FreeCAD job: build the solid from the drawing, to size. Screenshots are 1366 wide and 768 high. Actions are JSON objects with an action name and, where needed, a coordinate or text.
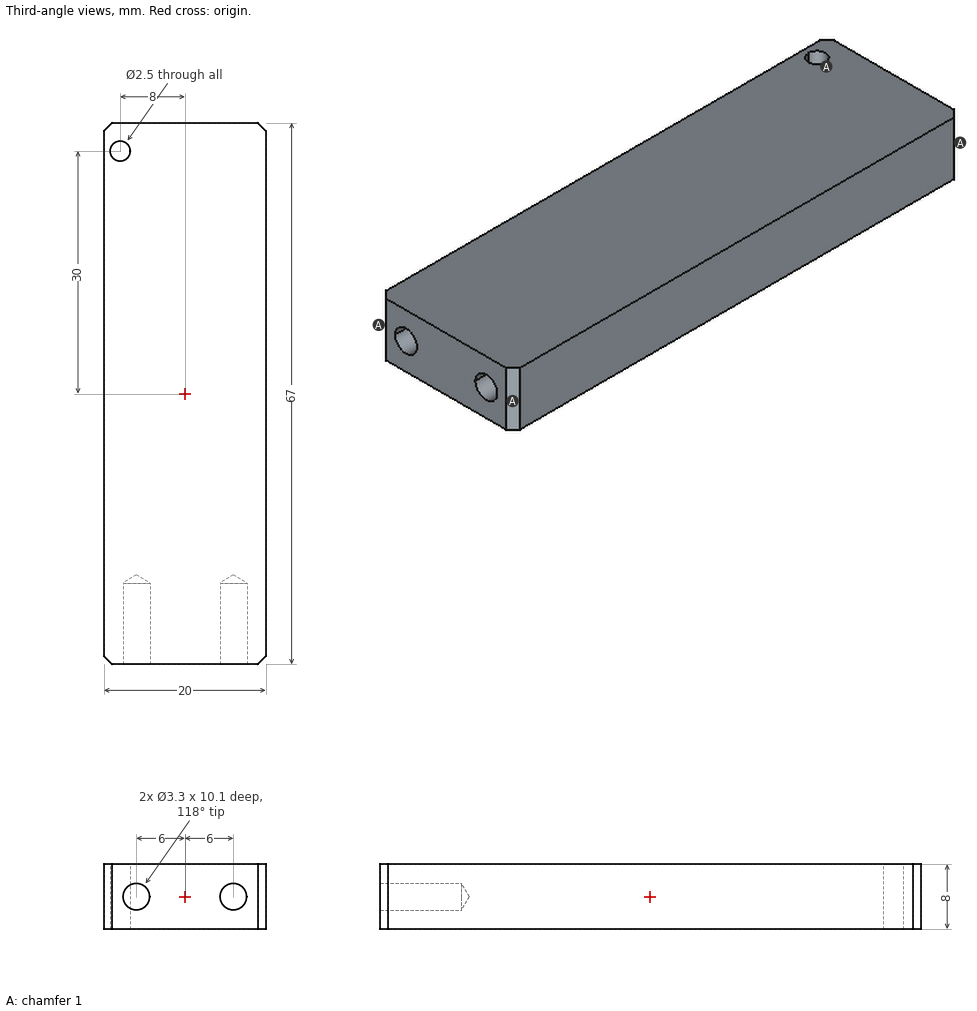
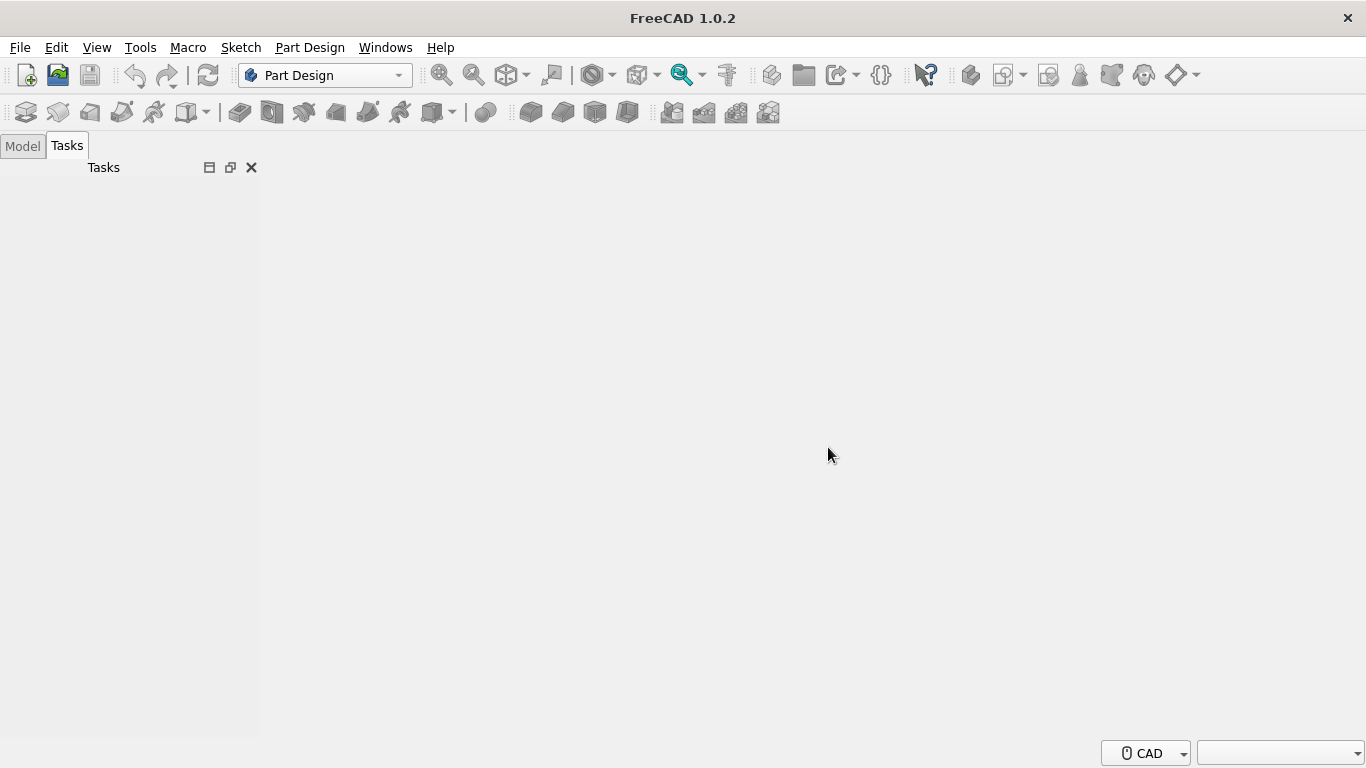
{"action": "key", "text": "ctrl+n"}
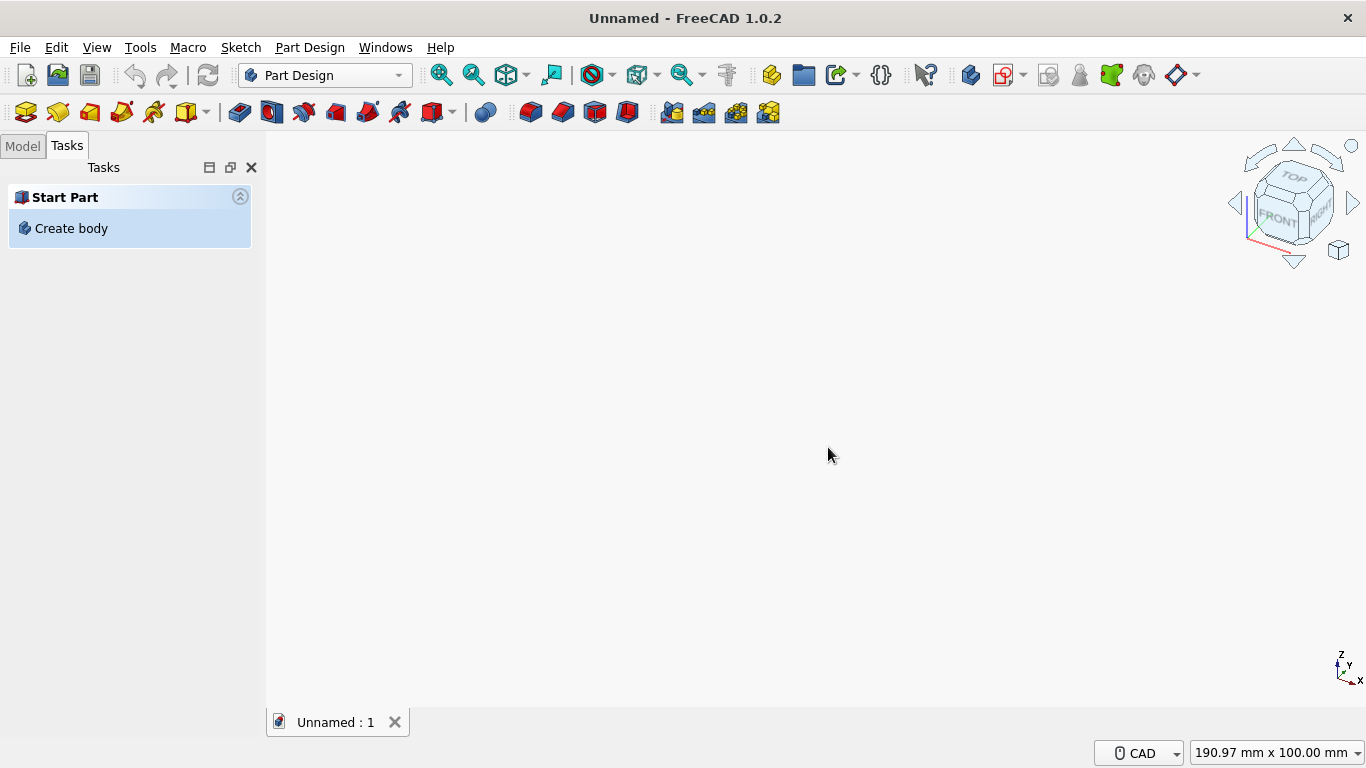
{"action": "left_click", "coordinate": [1004, 76]}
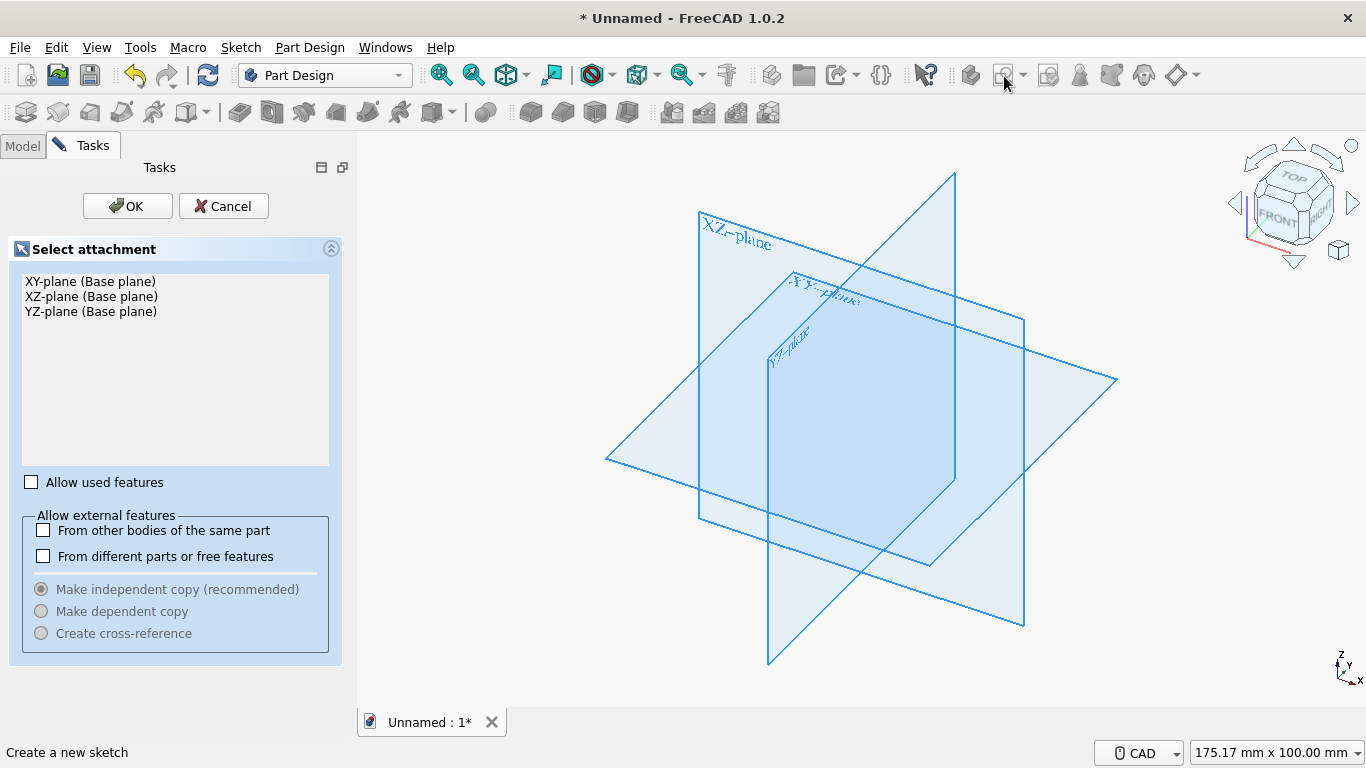
{"action": "left_click", "coordinate": [82, 282]}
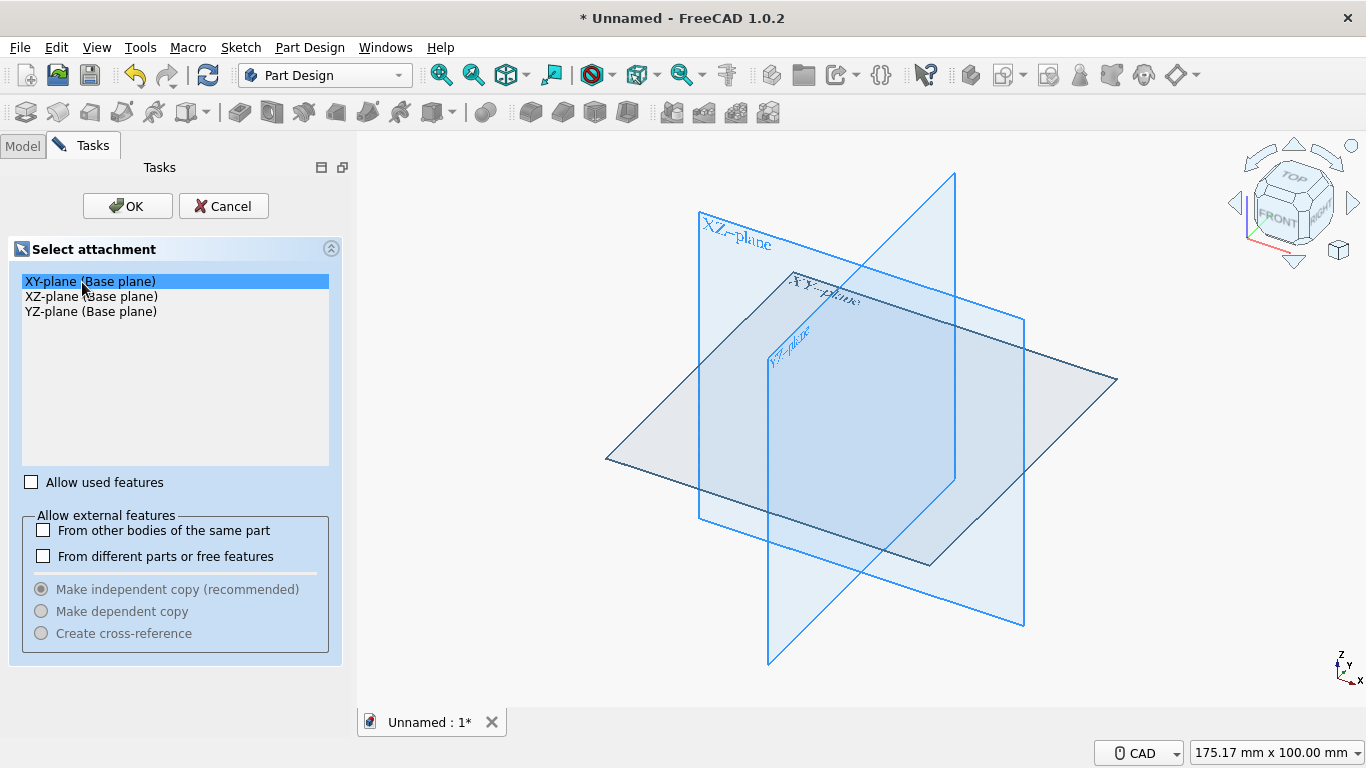
{"action": "left_click", "coordinate": [128, 206]}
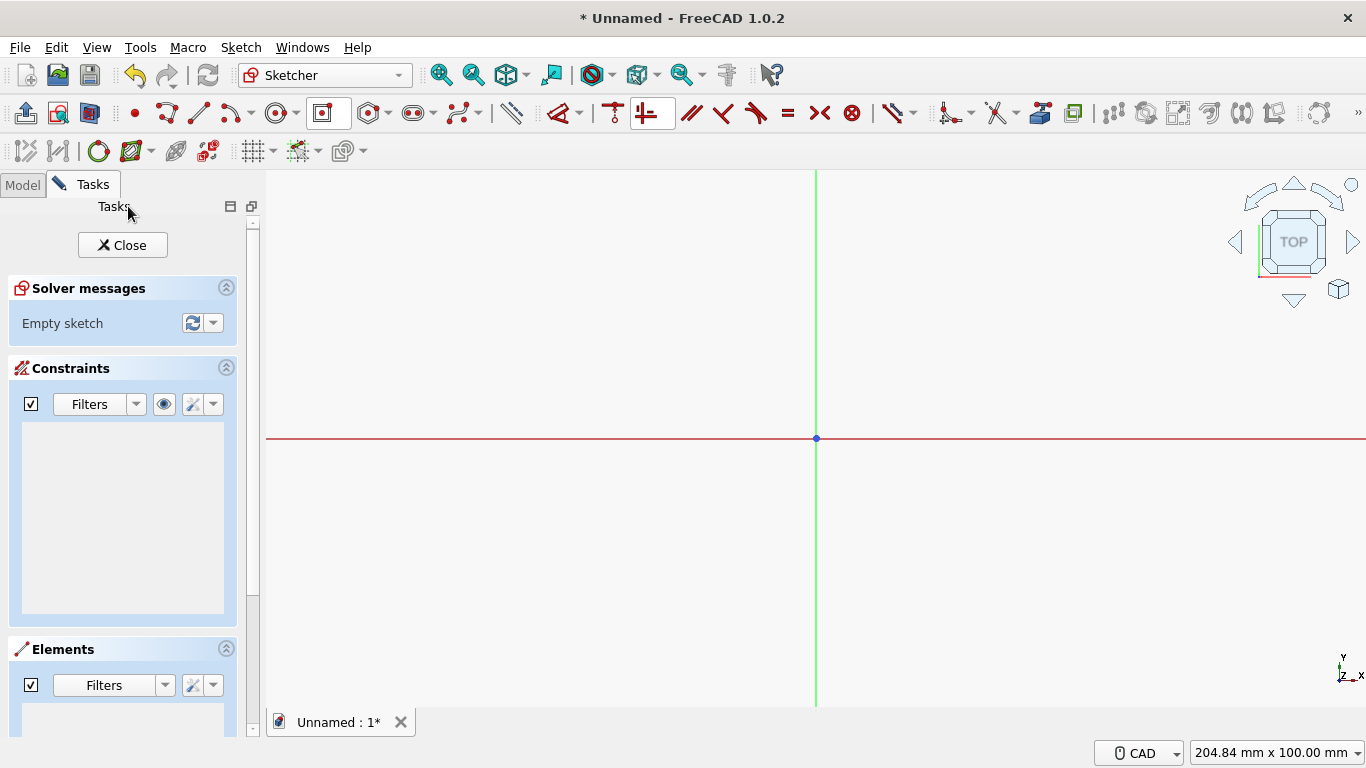
{"action": "key", "text": "g v"}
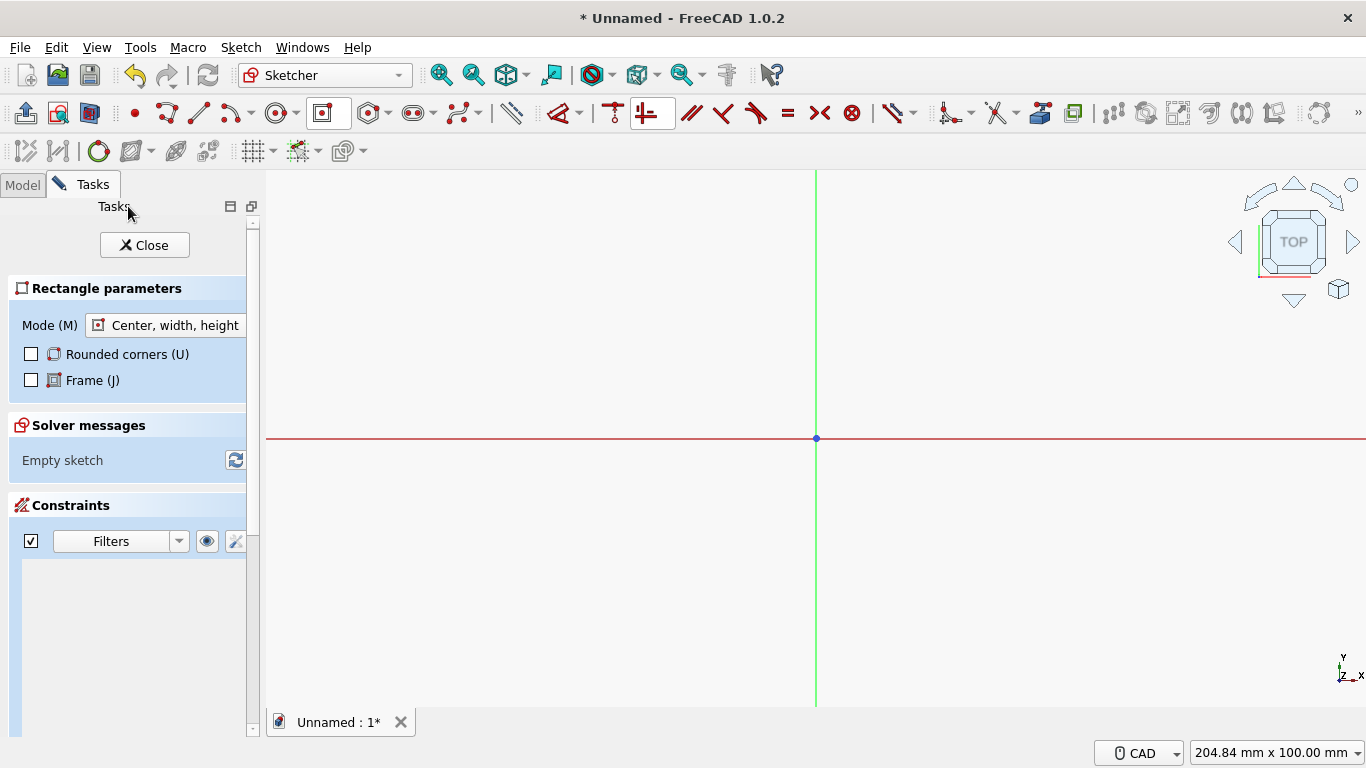
{"action": "left_click", "coordinate": [816, 438]}
{"action": "mouse_move", "coordinate": [870, 259]}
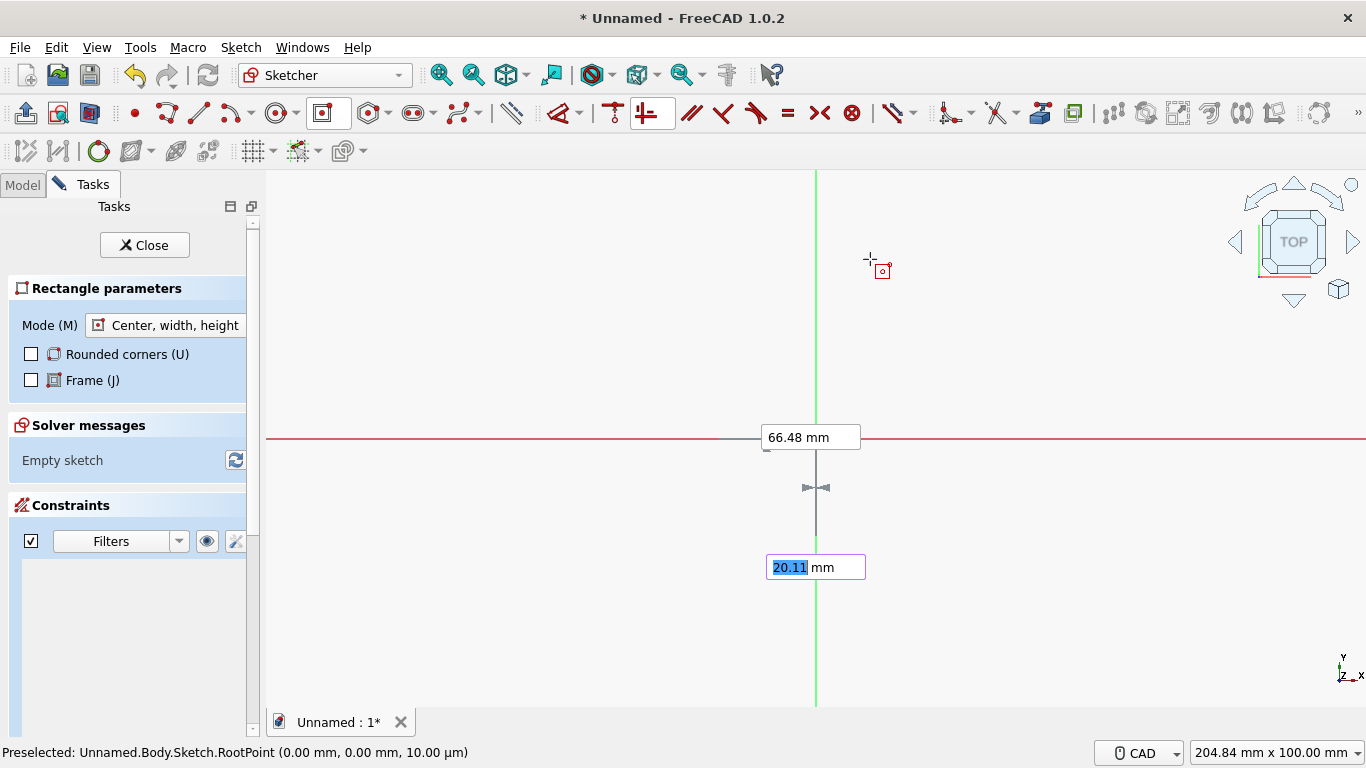
{"action": "type", "text": "20"}
{"action": "key", "text": "Tab"}
{"action": "type", "text": "67"}
{"action": "key", "text": "Return"}
{"action": "key", "text": "Escape"}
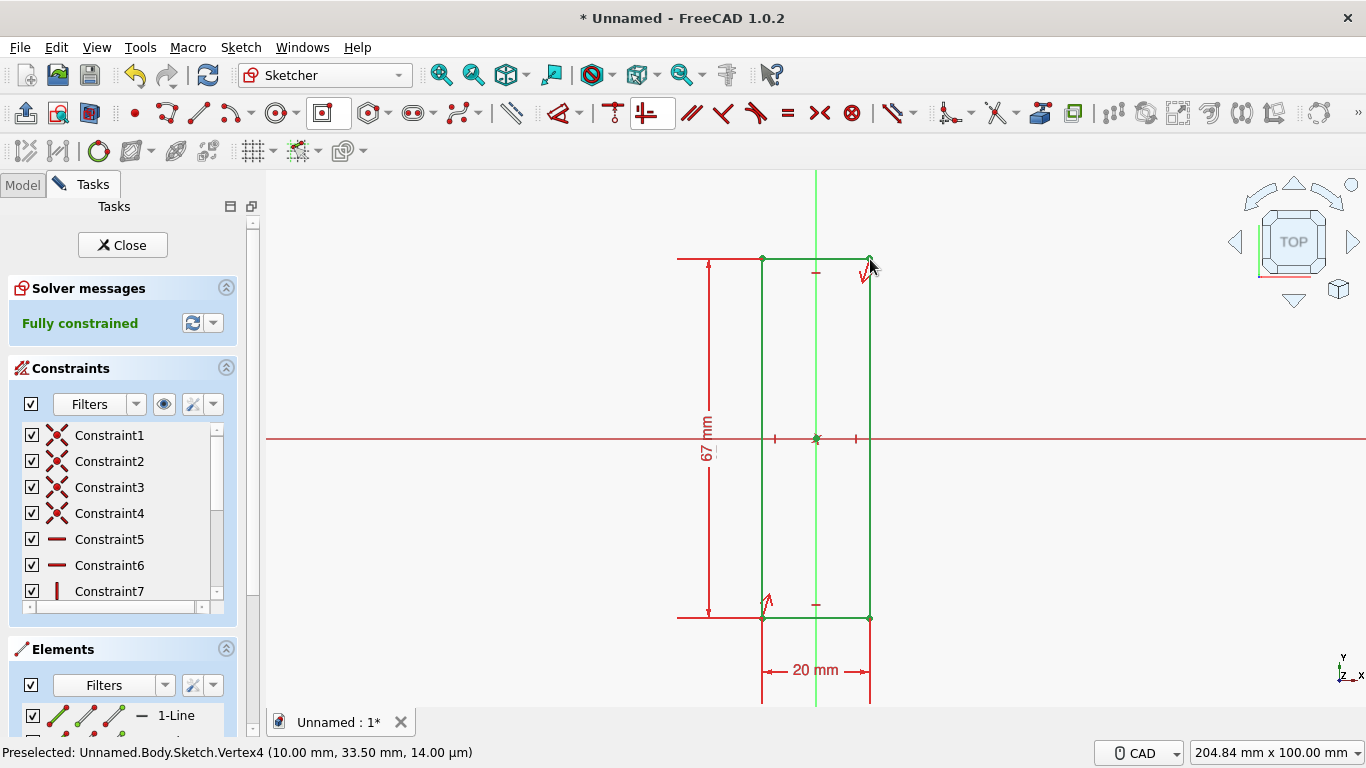
{"action": "left_click", "coordinate": [123, 245]}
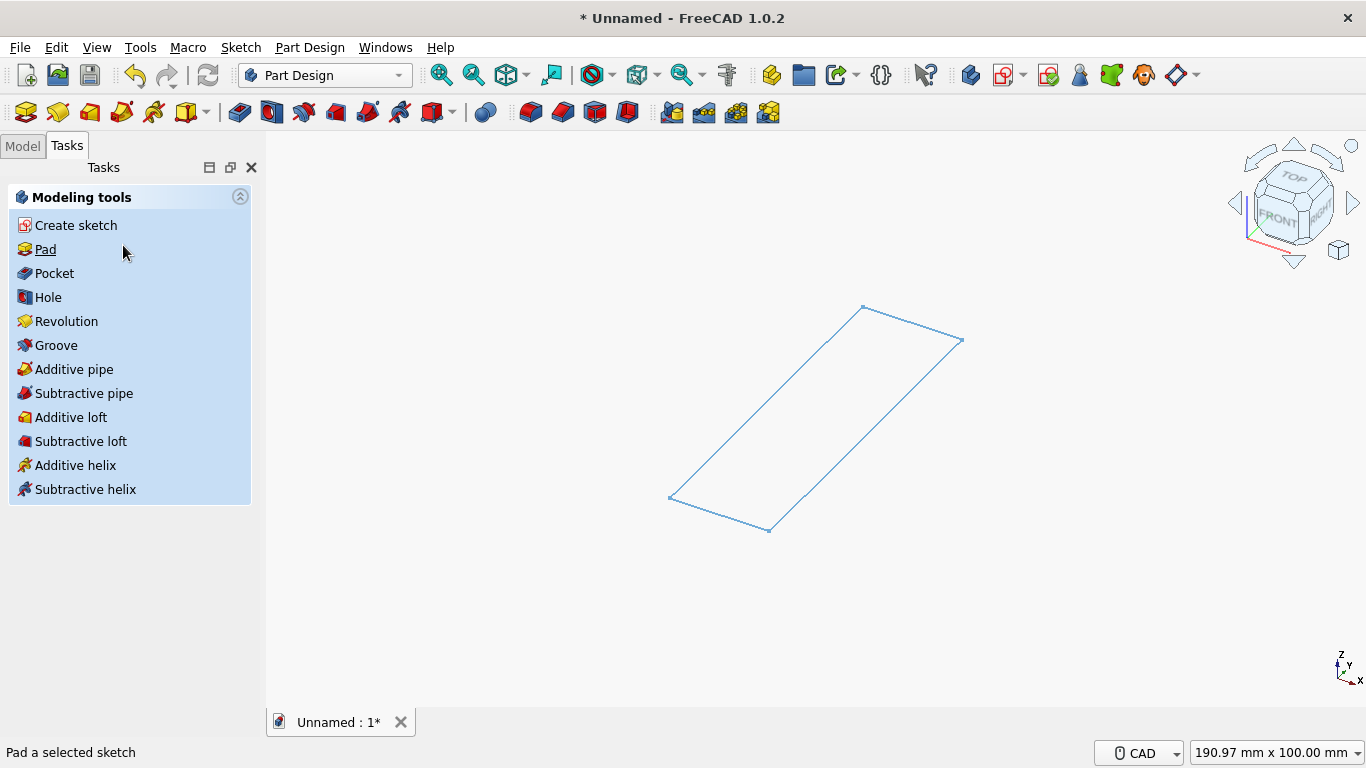
{"action": "left_click", "coordinate": [26, 112]}